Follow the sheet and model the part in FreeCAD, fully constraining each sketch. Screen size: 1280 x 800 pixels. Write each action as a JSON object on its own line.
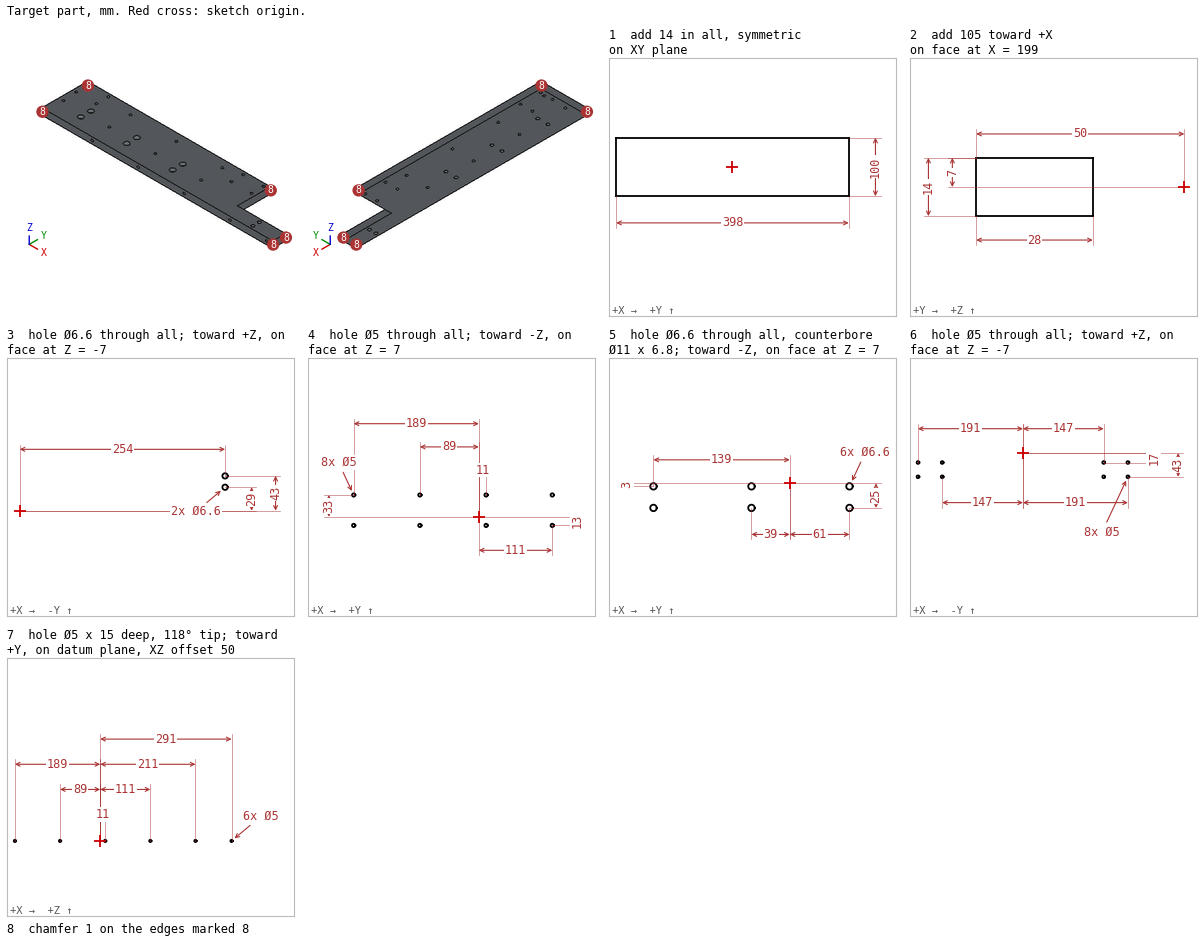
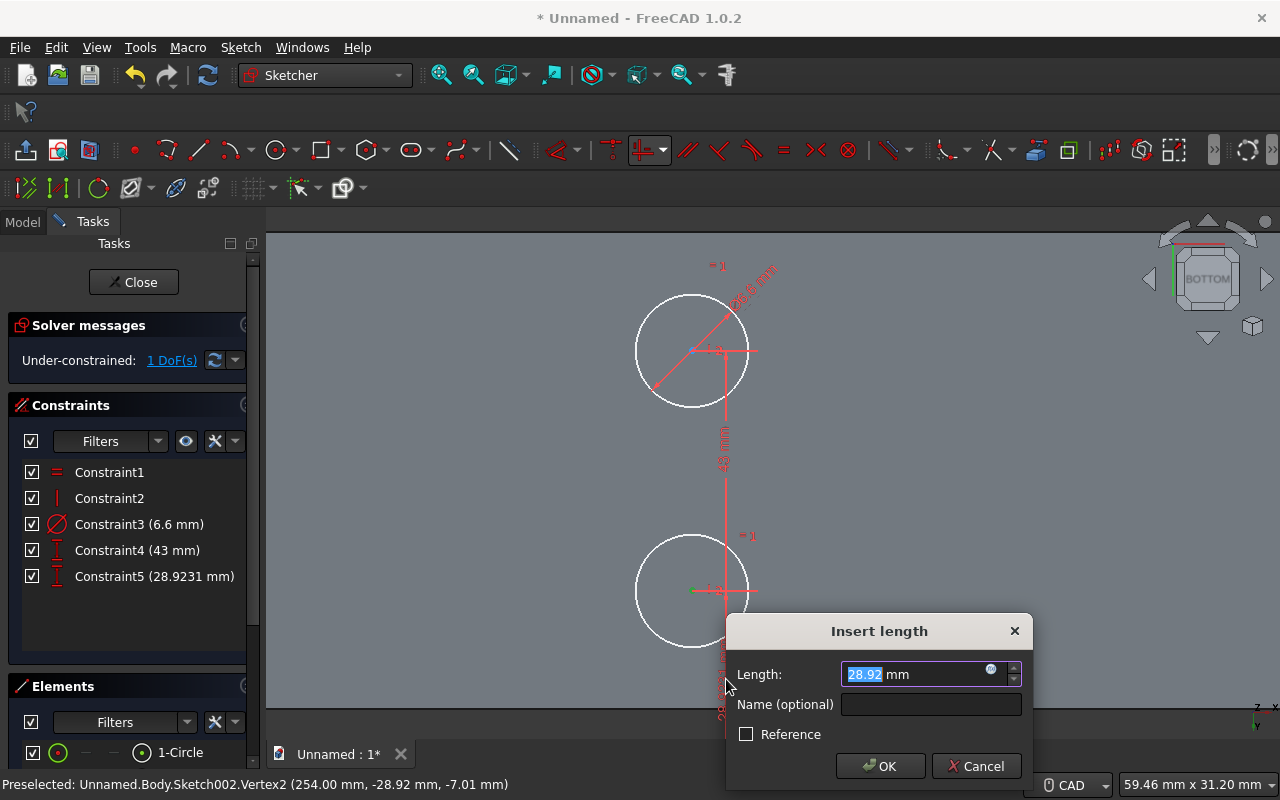
{"action": "type", "text": "29"}
{"action": "key", "text": "Return"}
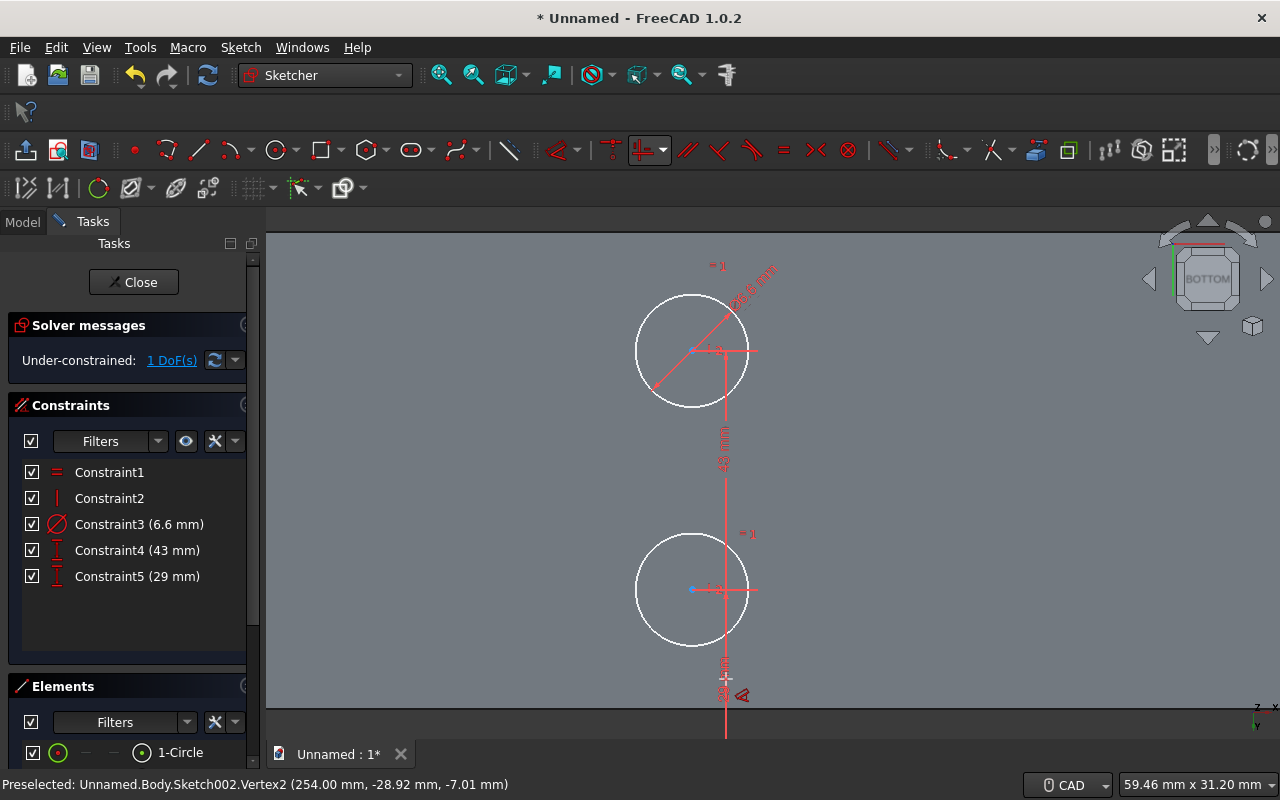
{"action": "left_click", "coordinate": [692, 351]}
{"action": "left_click", "coordinate": [493, 317]}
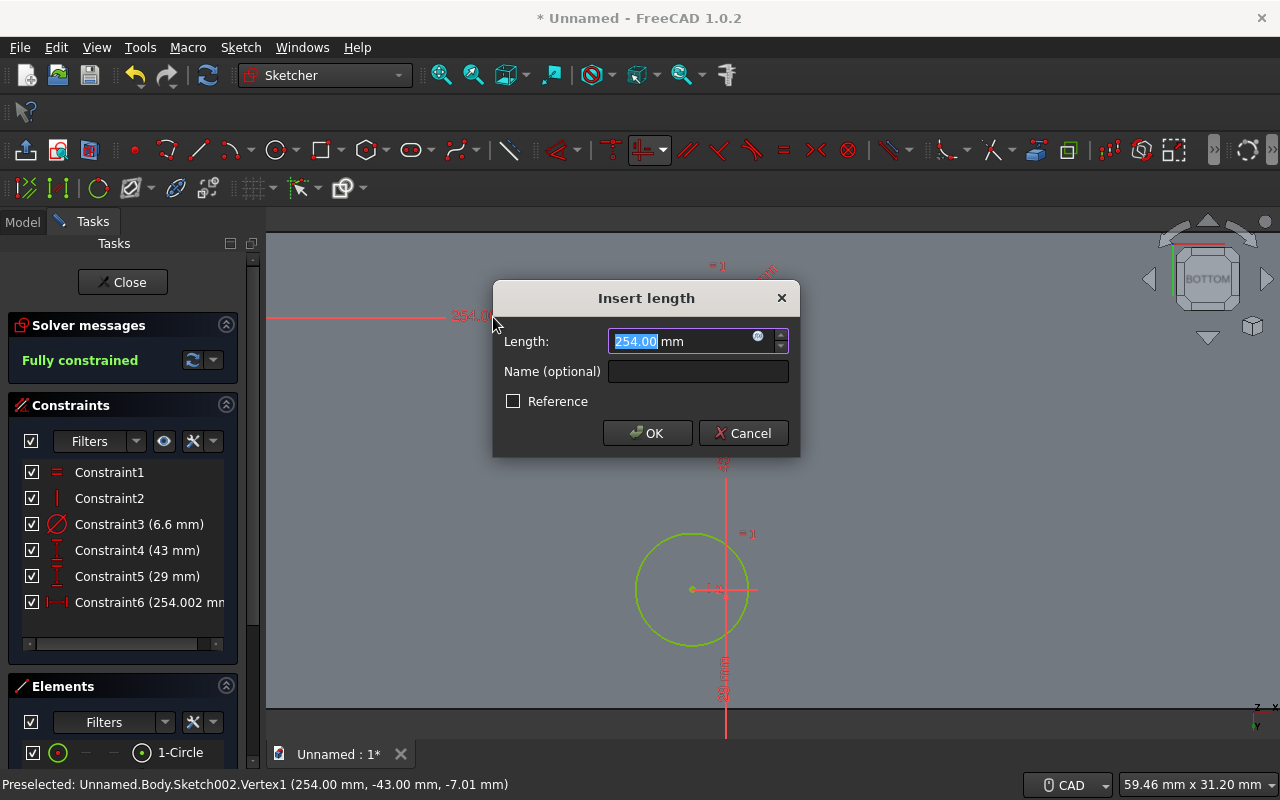
{"action": "type", "text": "254"}
{"action": "key", "text": "Return"}
{"action": "key", "text": "Escape"}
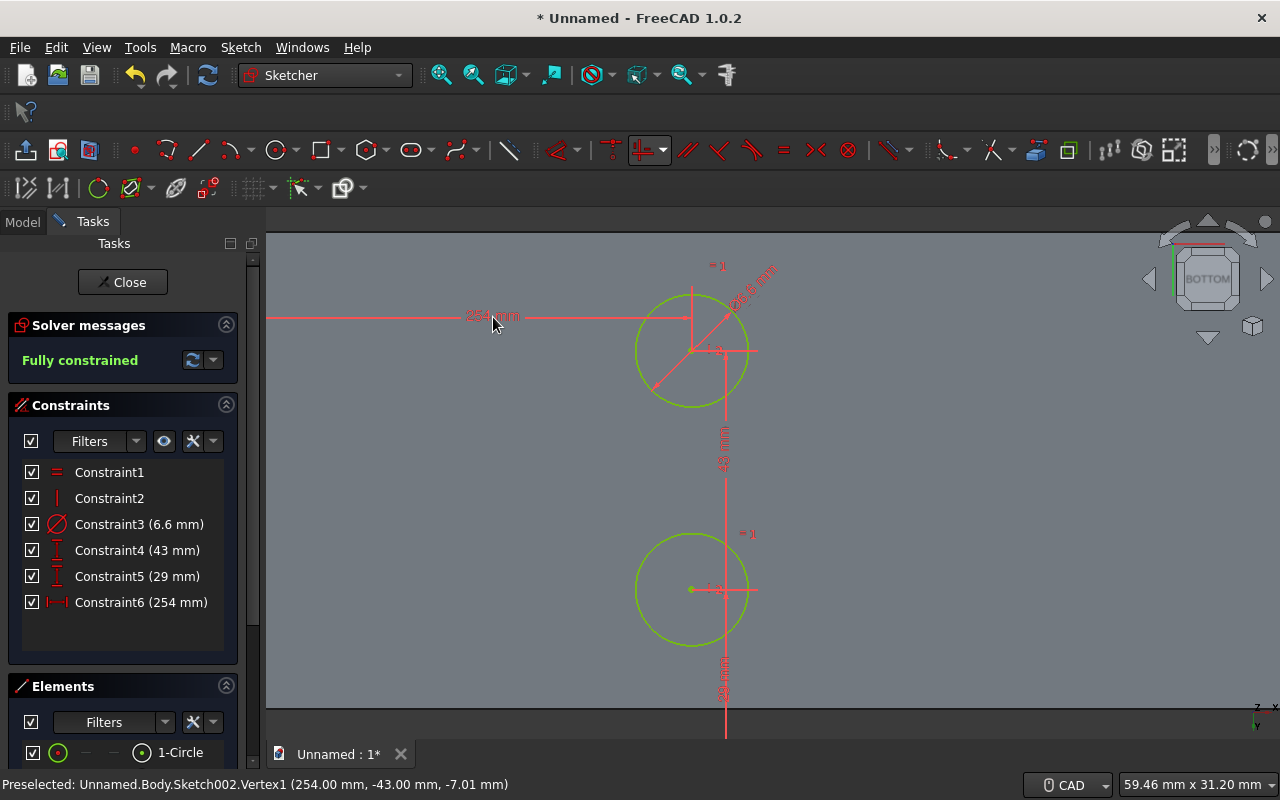
{"action": "left_click", "coordinate": [123, 282]}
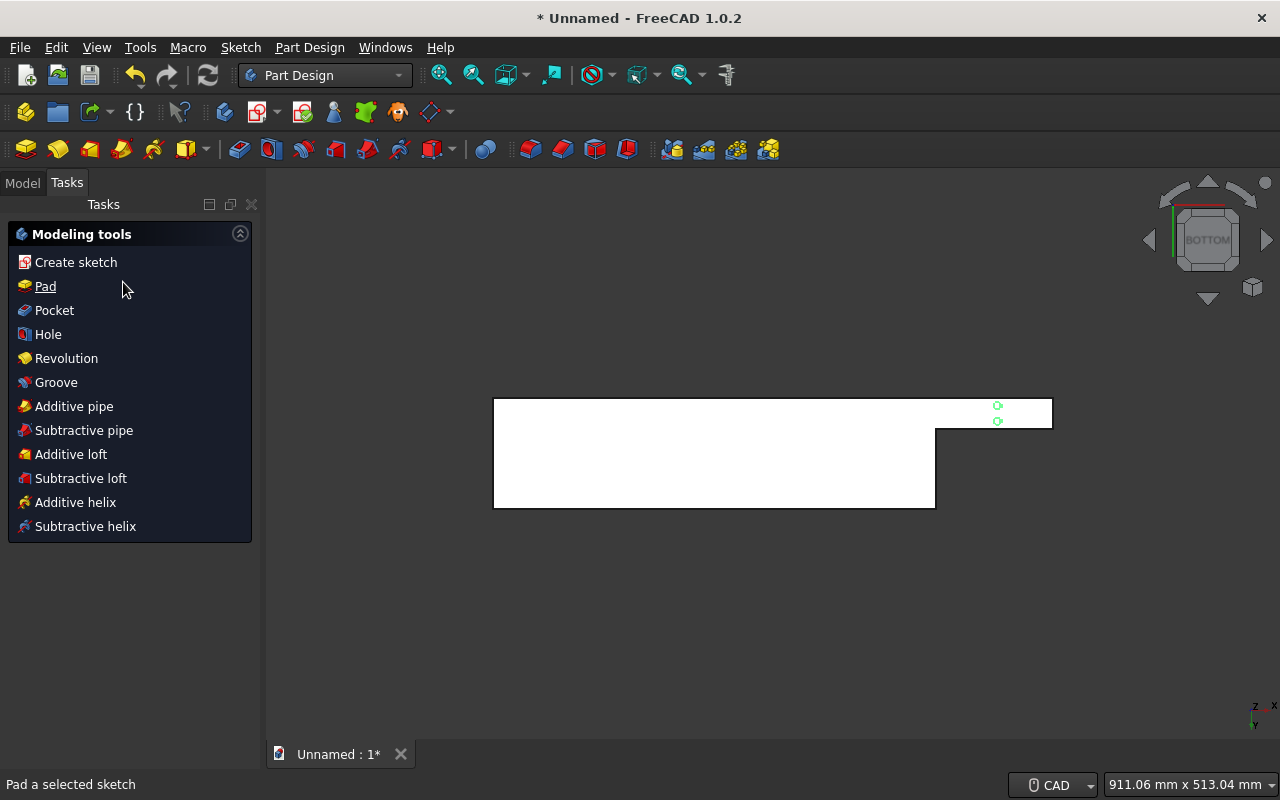
{"action": "left_click", "coordinate": [272, 150]}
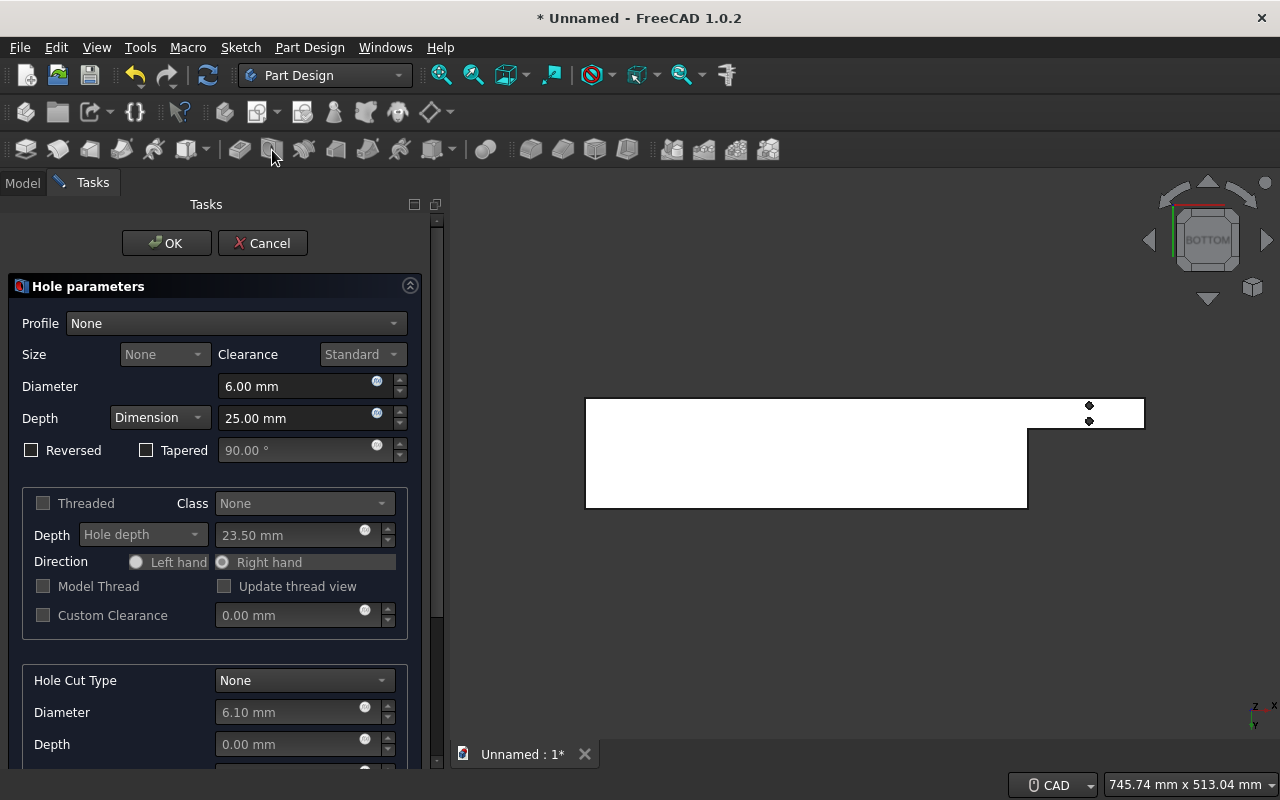
{"action": "triple_click", "coordinate": [305, 386]}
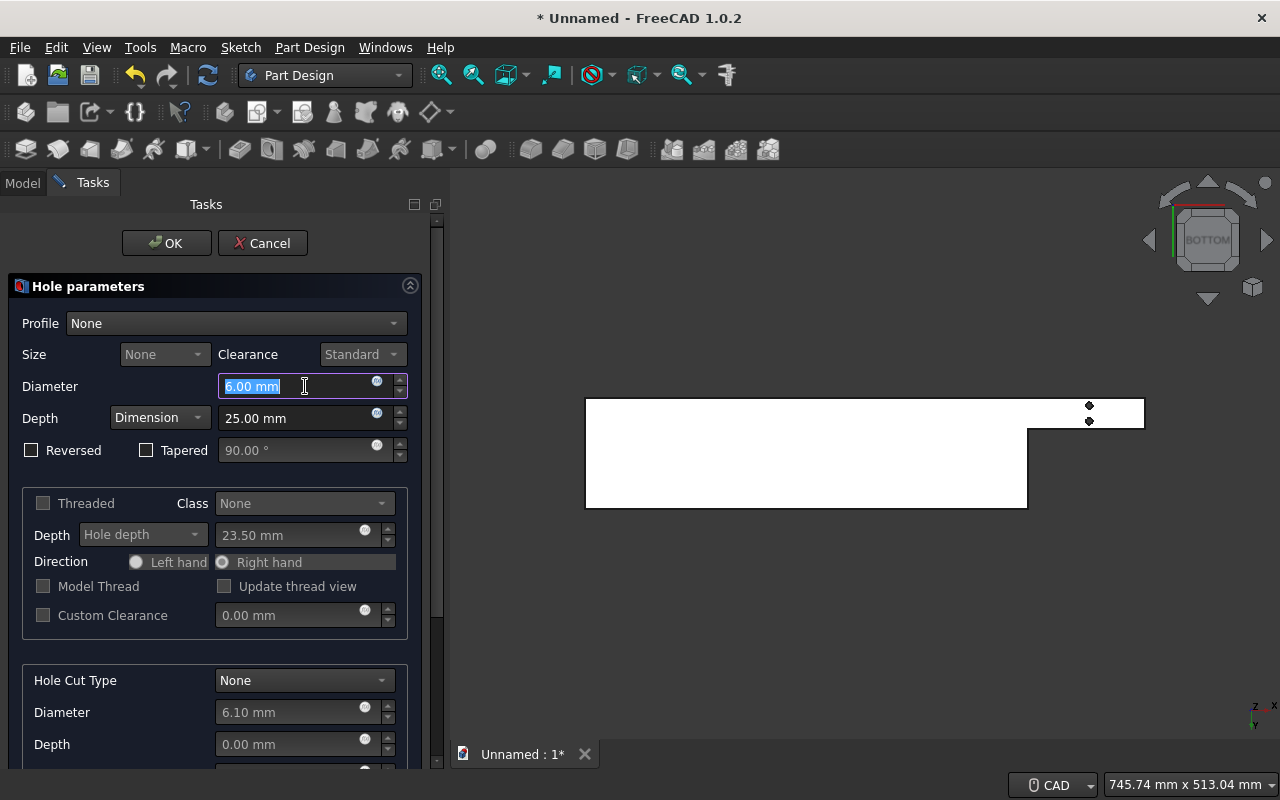
{"action": "type", "text": "6.6"}
{"action": "key", "text": "Tab"}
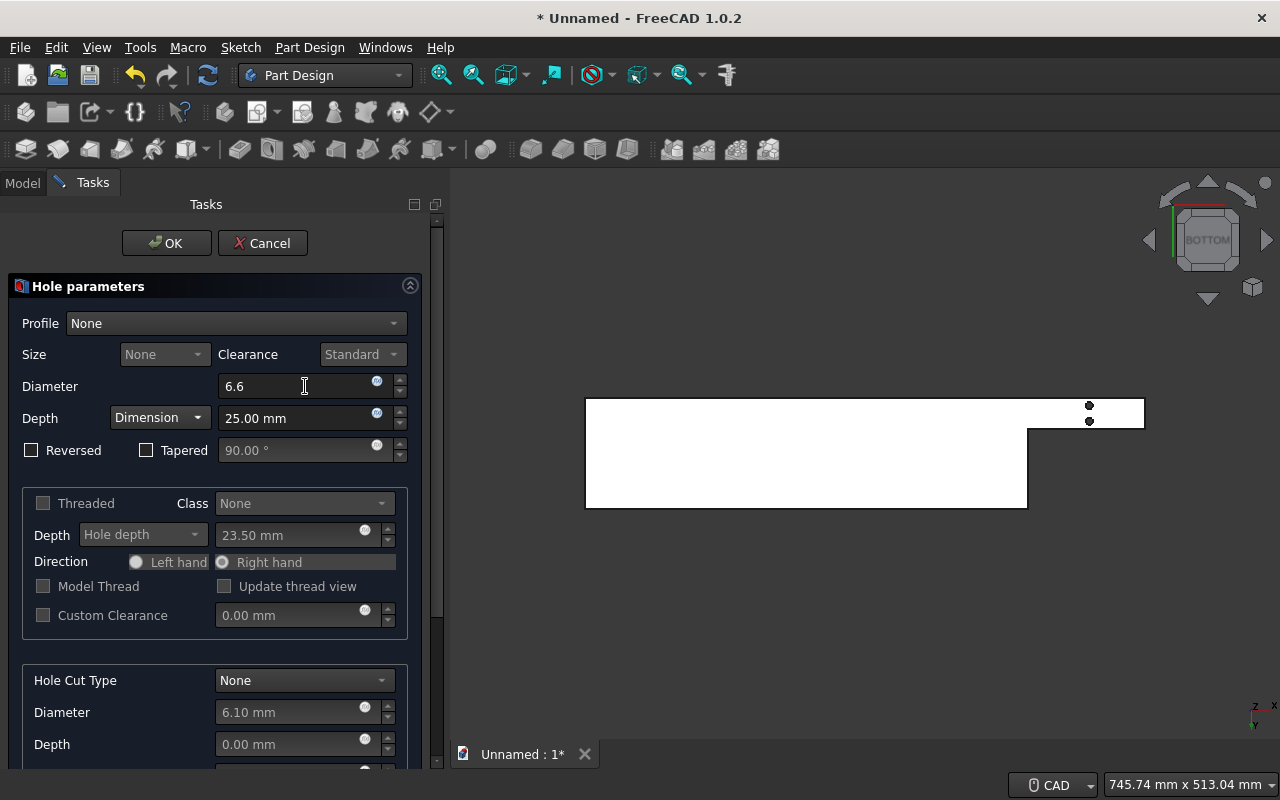
{"action": "left_click", "coordinate": [161, 418]}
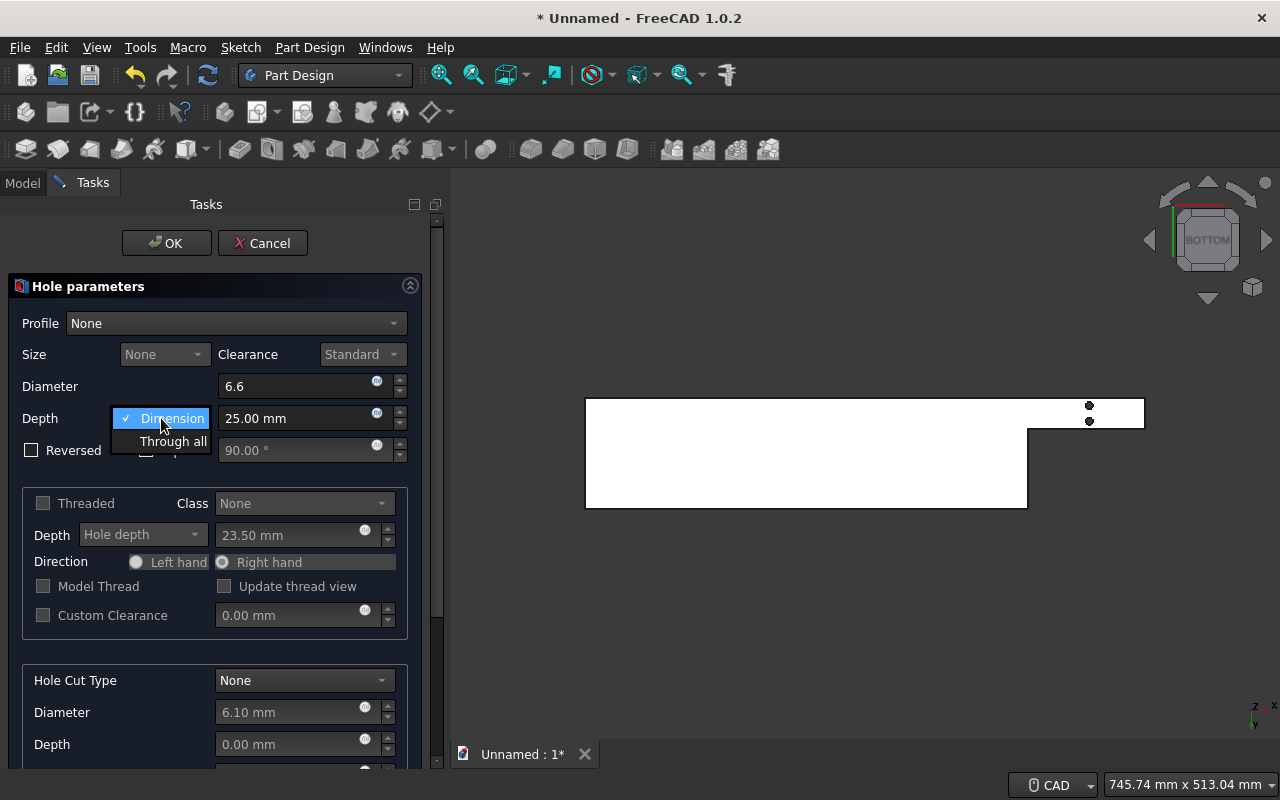
{"action": "left_click", "coordinate": [160, 442]}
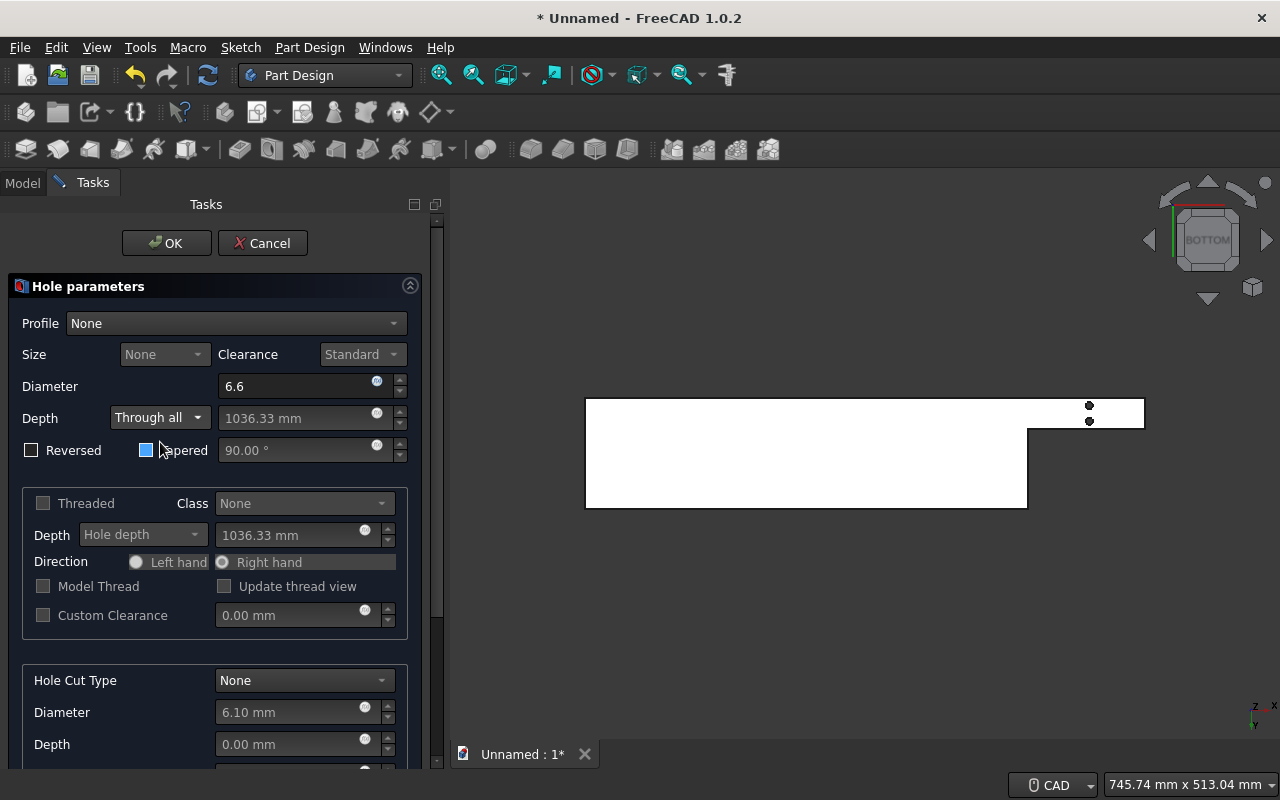
{"action": "left_click", "coordinate": [167, 243]}